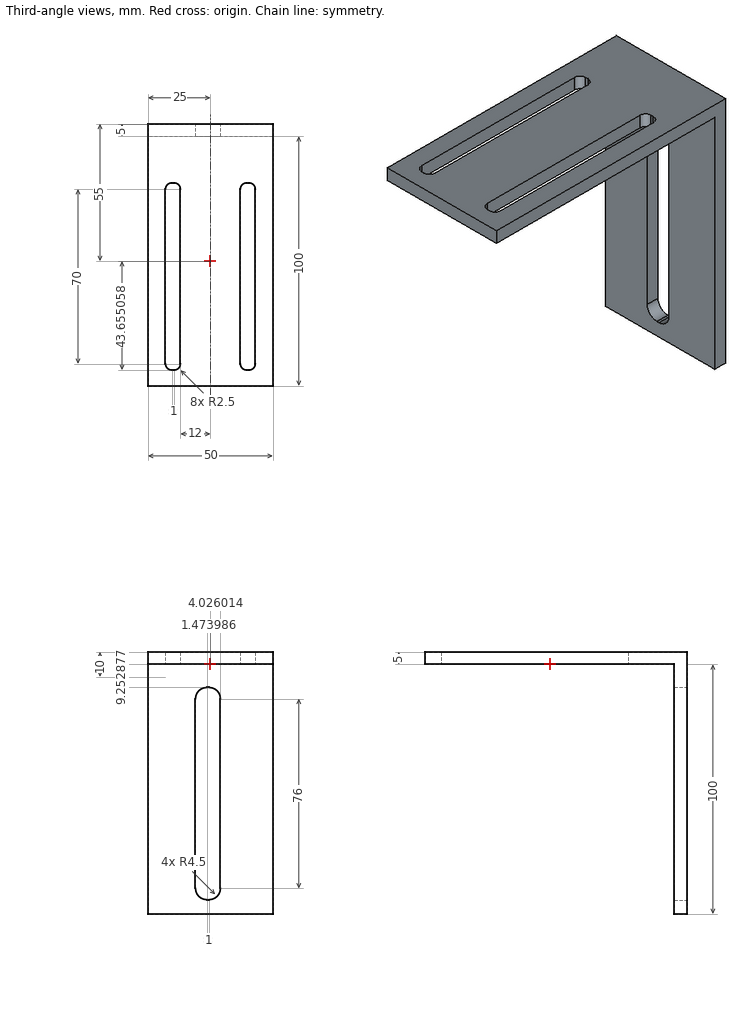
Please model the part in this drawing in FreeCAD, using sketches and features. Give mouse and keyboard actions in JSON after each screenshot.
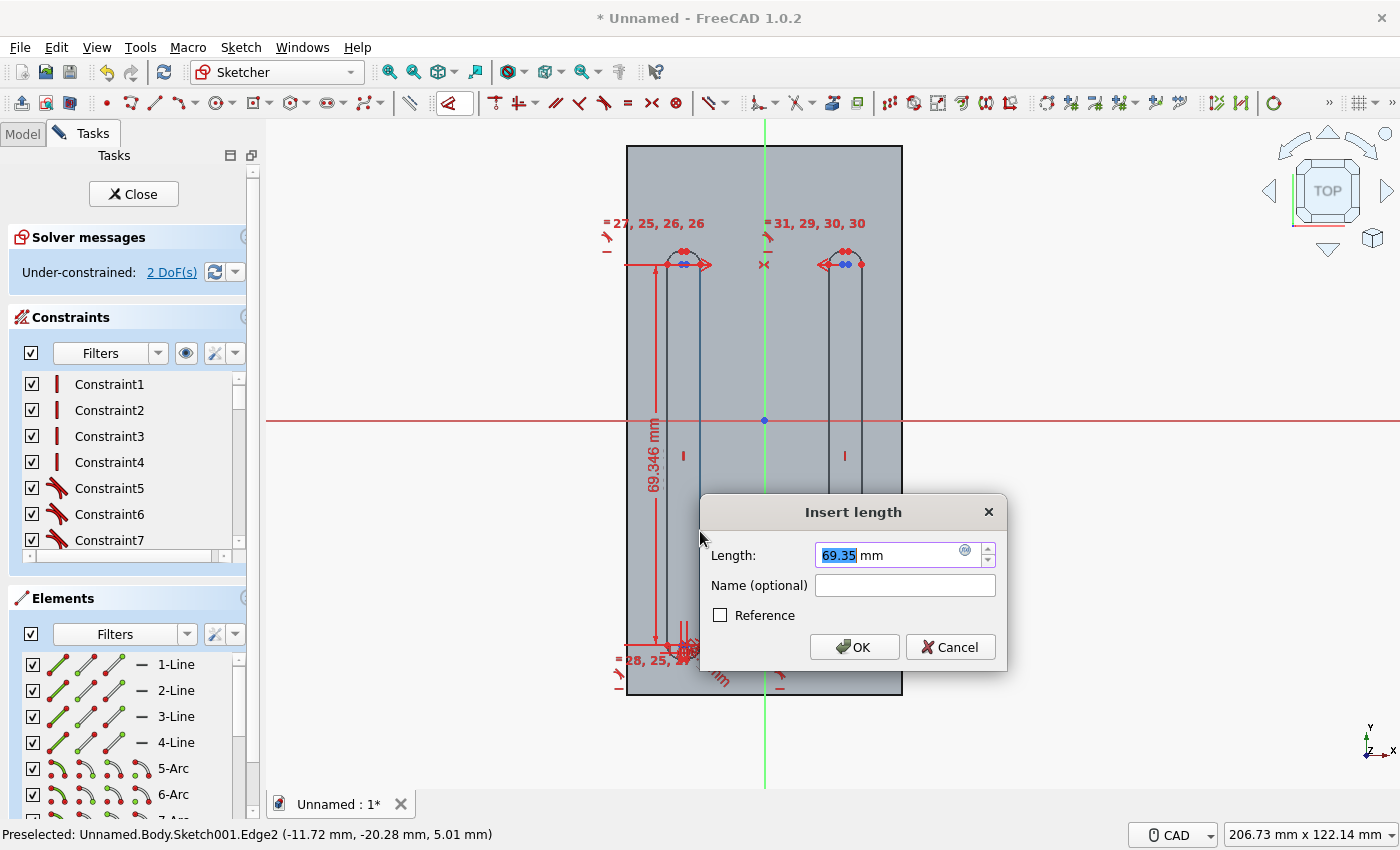
{"action": "type", "text": "70"}
{"action": "key", "text": "Return"}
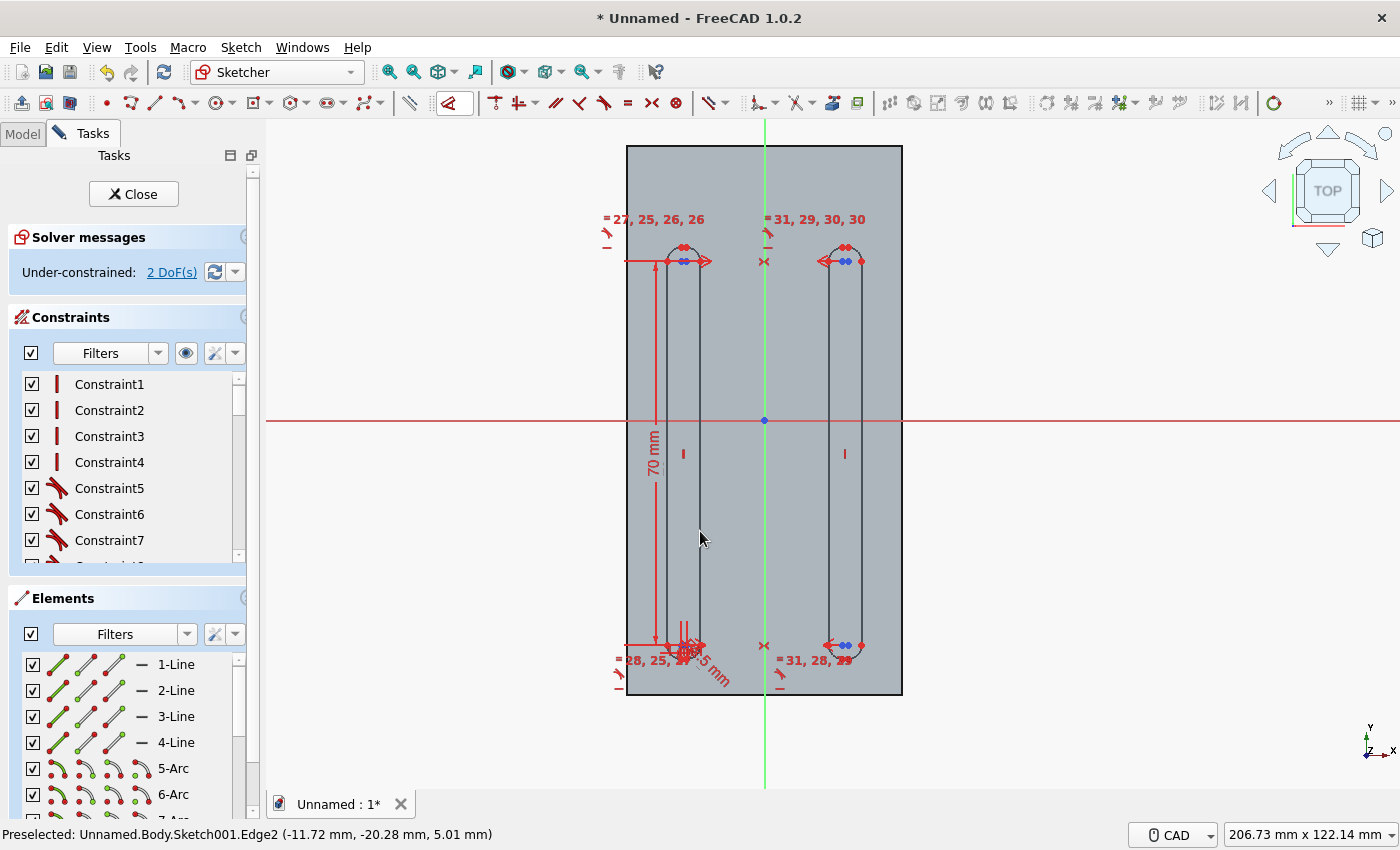
{"action": "left_click", "coordinate": [700, 645]}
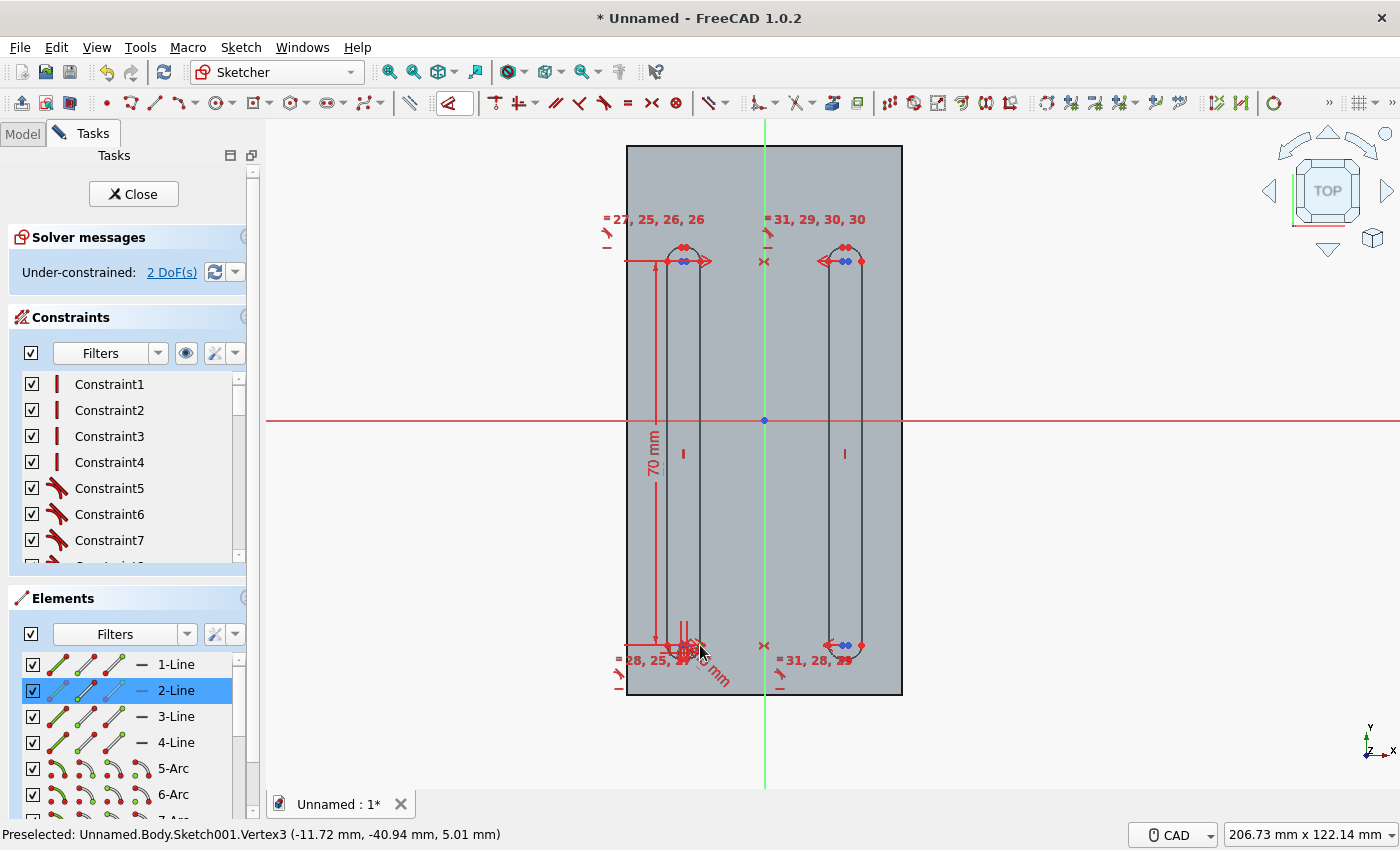
{"action": "key", "text": "l"}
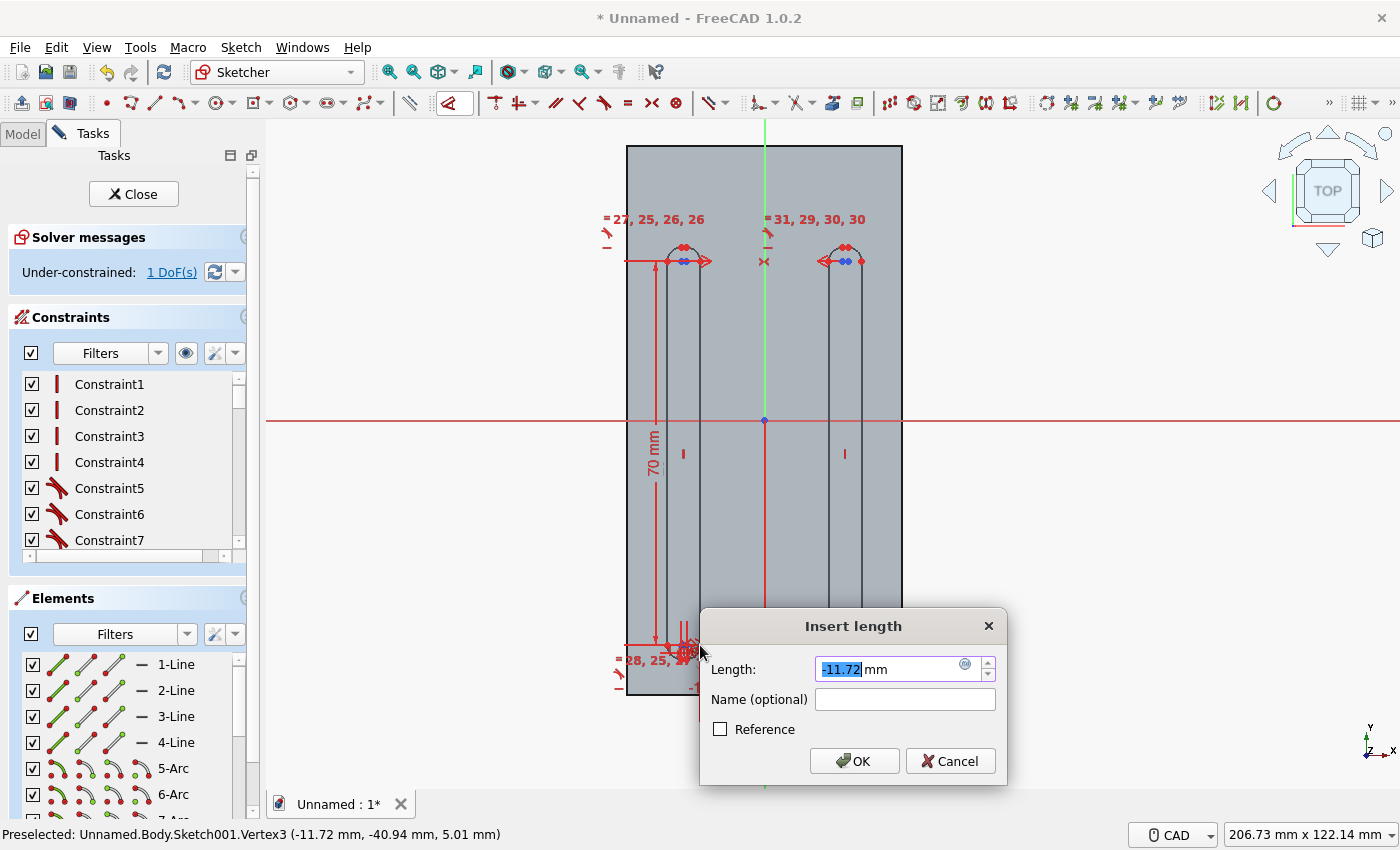
{"action": "type", "text": "-12"}
{"action": "key", "text": "Return"}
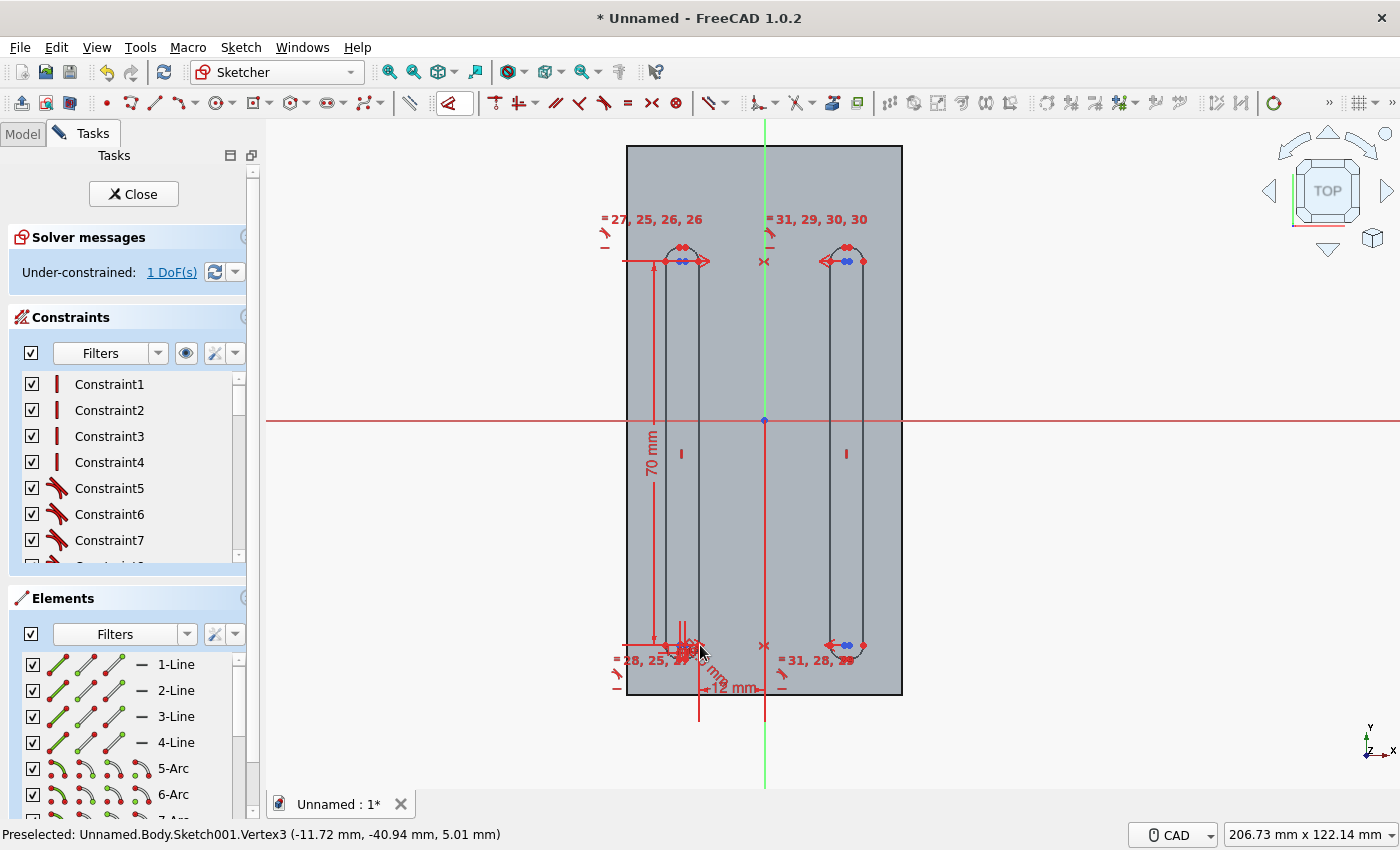
{"action": "scroll", "coordinate": [680, 659], "scroll_direction": "up", "scroll_amount": 5}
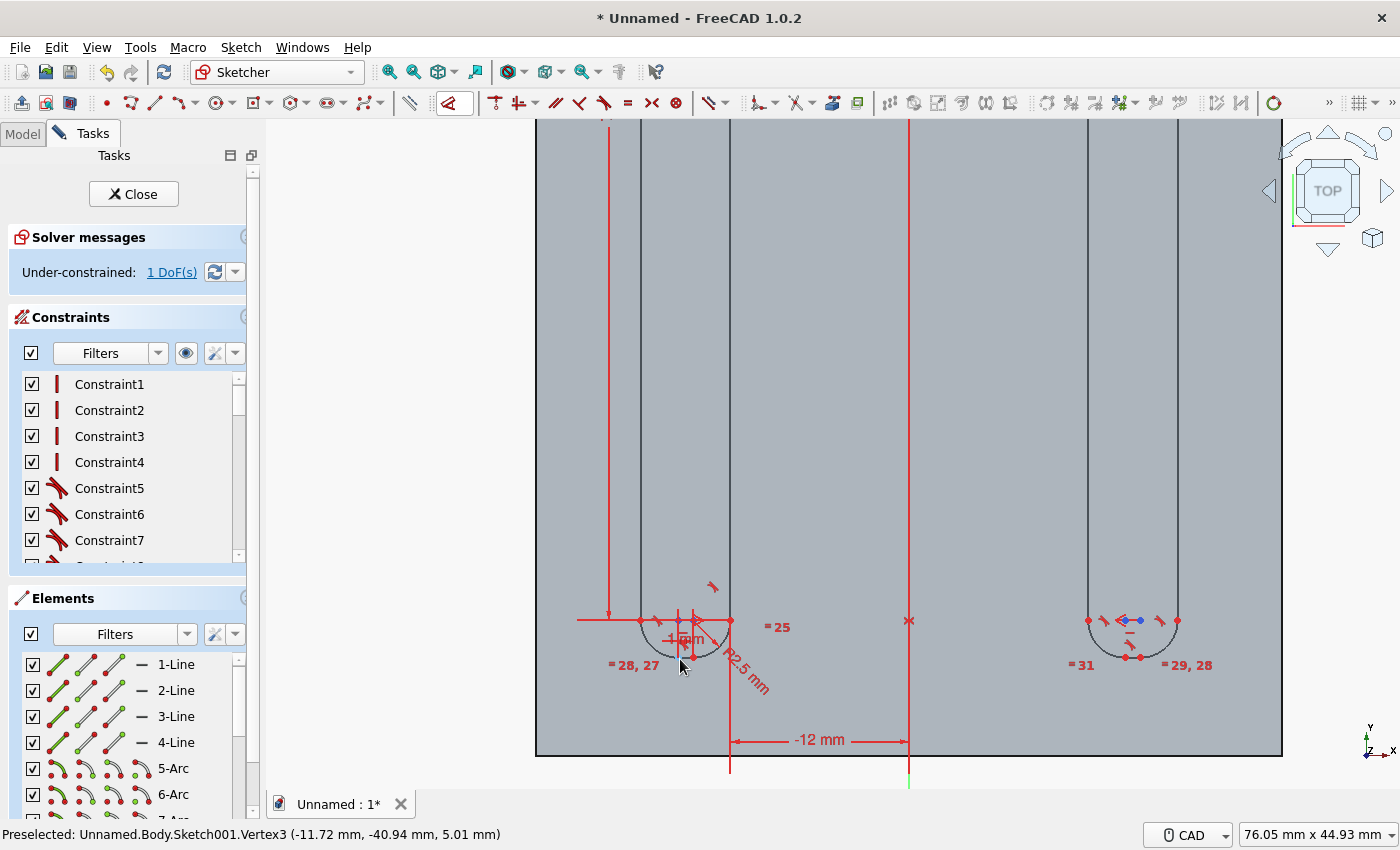
{"action": "left_click", "coordinate": [678, 658]}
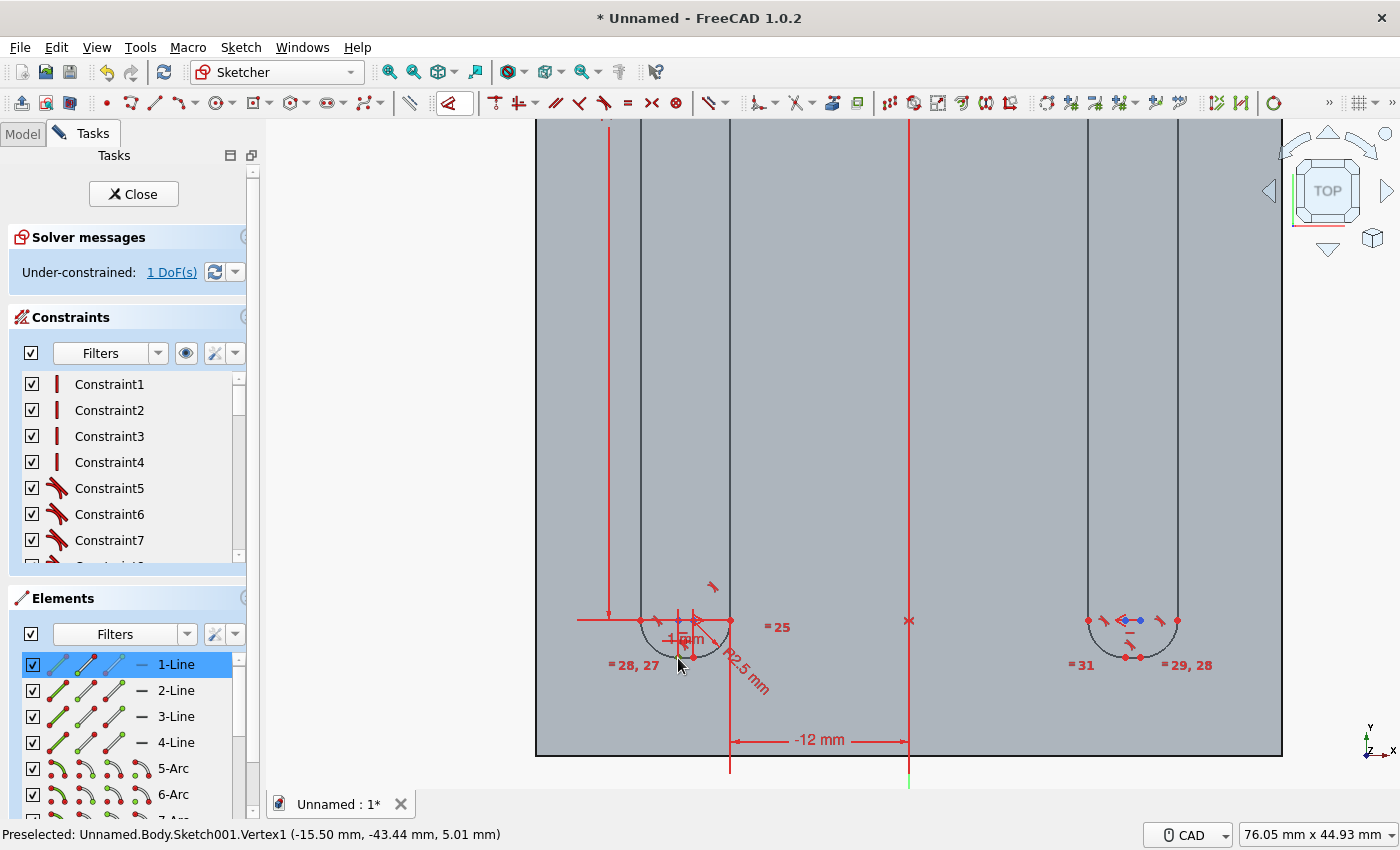
{"action": "key", "text": "i"}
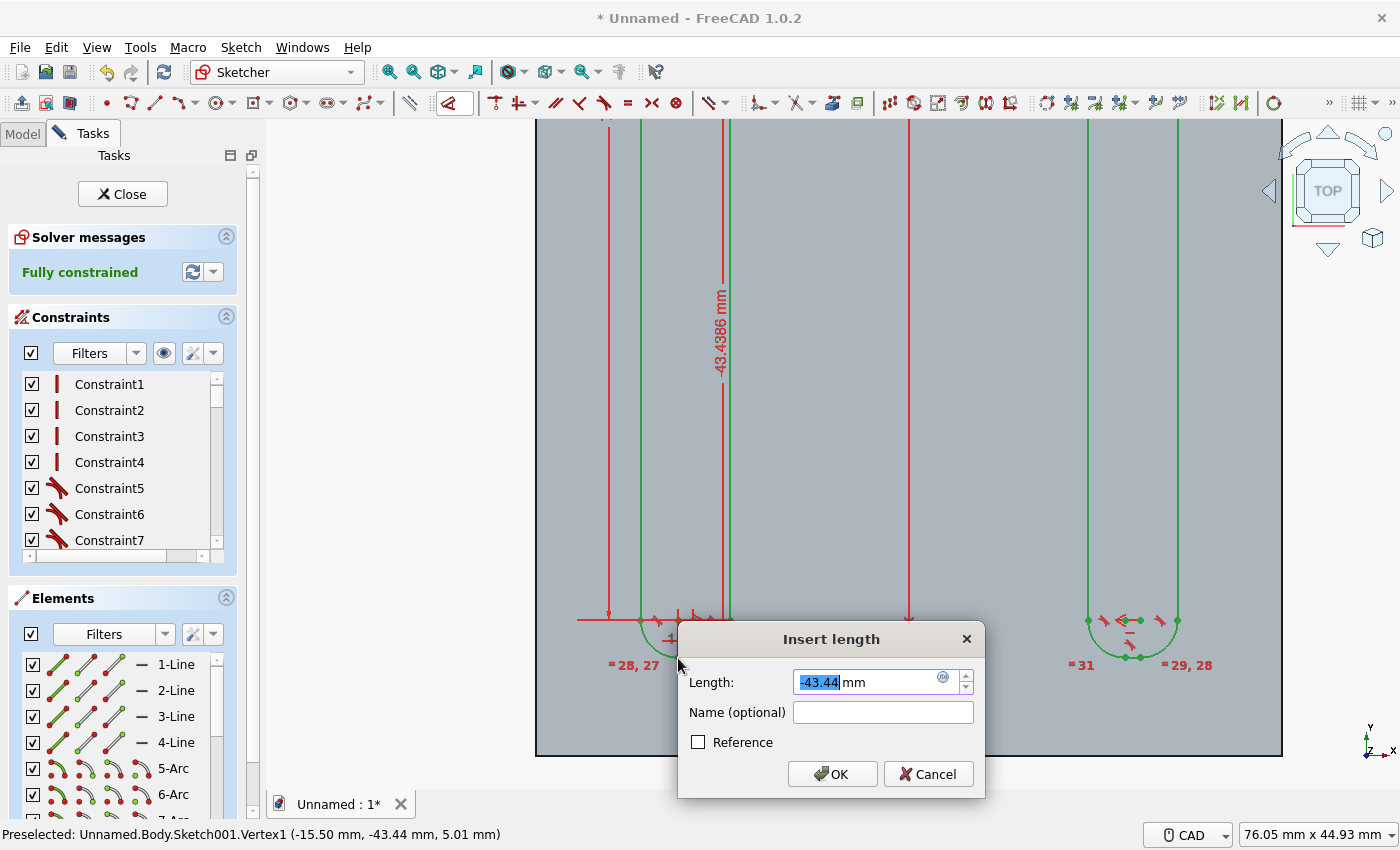
{"action": "type", "text": "-43.655058"}
{"action": "key", "text": "Return"}